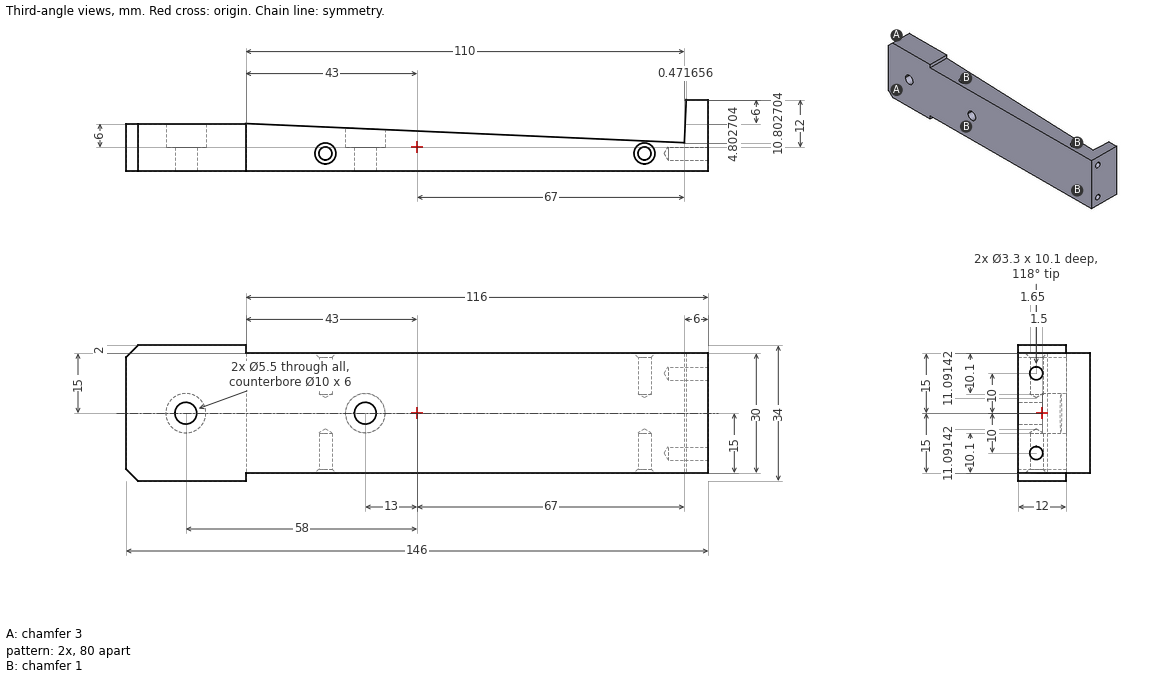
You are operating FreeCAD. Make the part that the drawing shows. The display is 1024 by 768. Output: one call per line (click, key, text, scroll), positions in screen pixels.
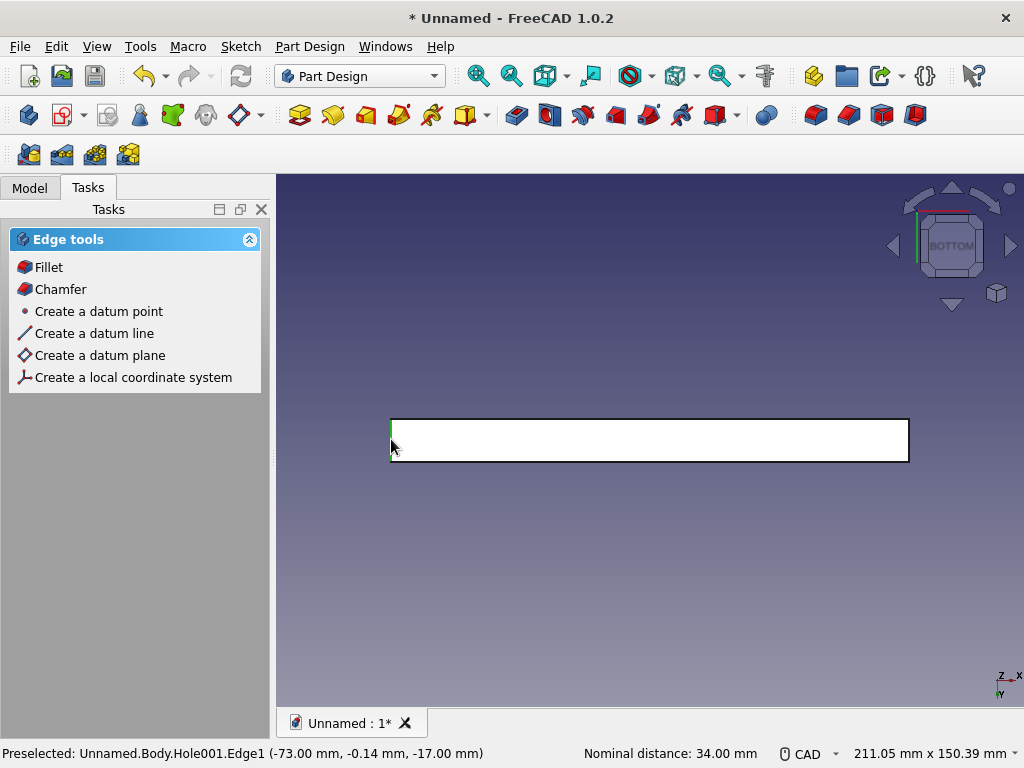
click(849, 116)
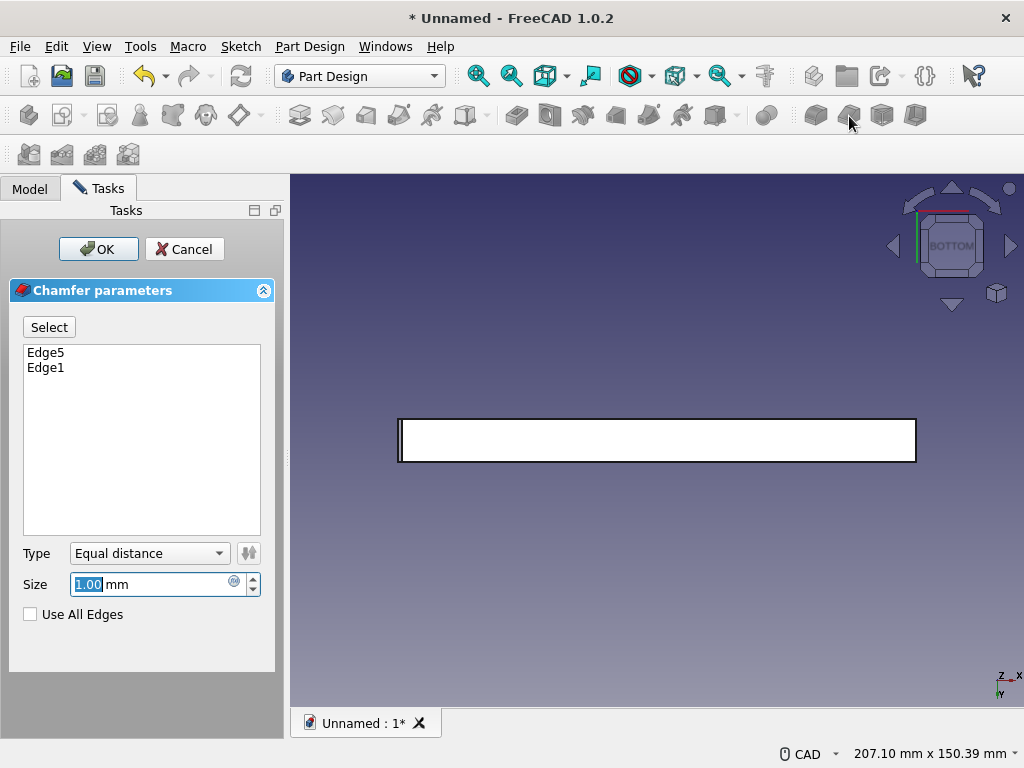
text(3)
key(Tab)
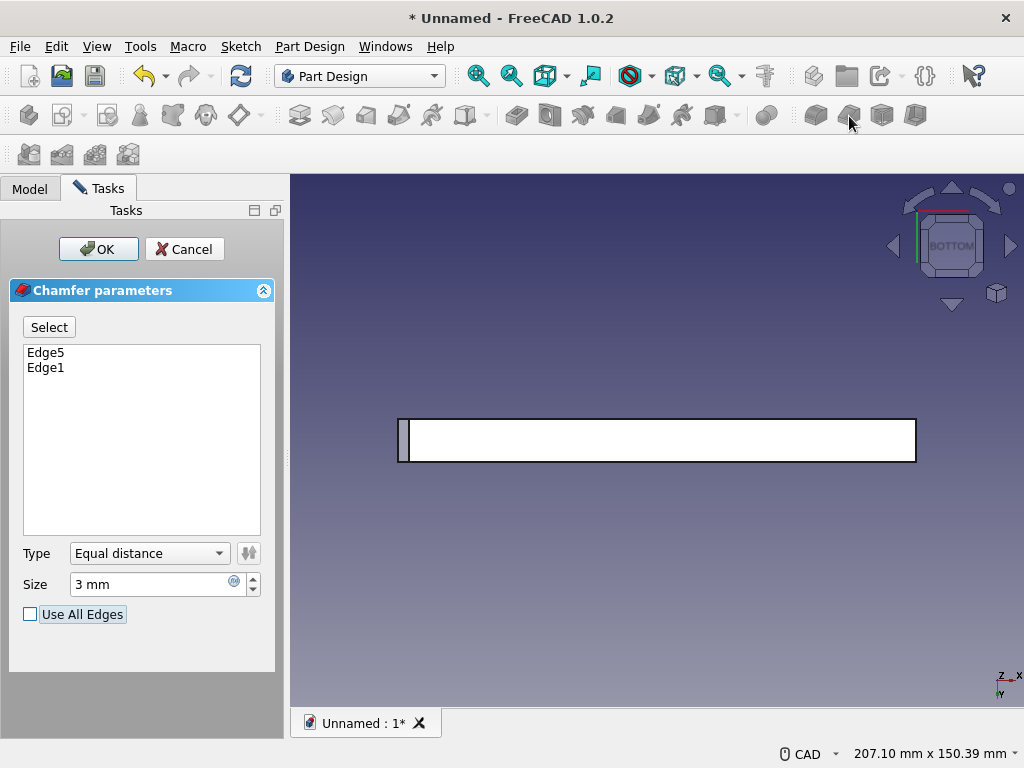
click(99, 249)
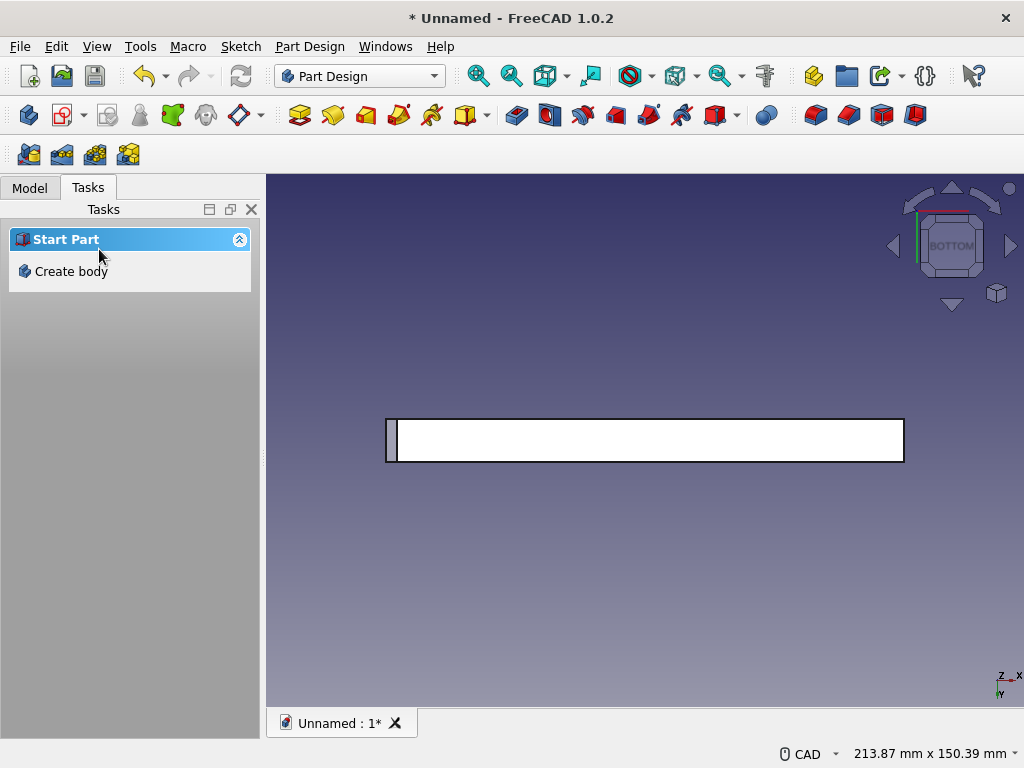
key(4)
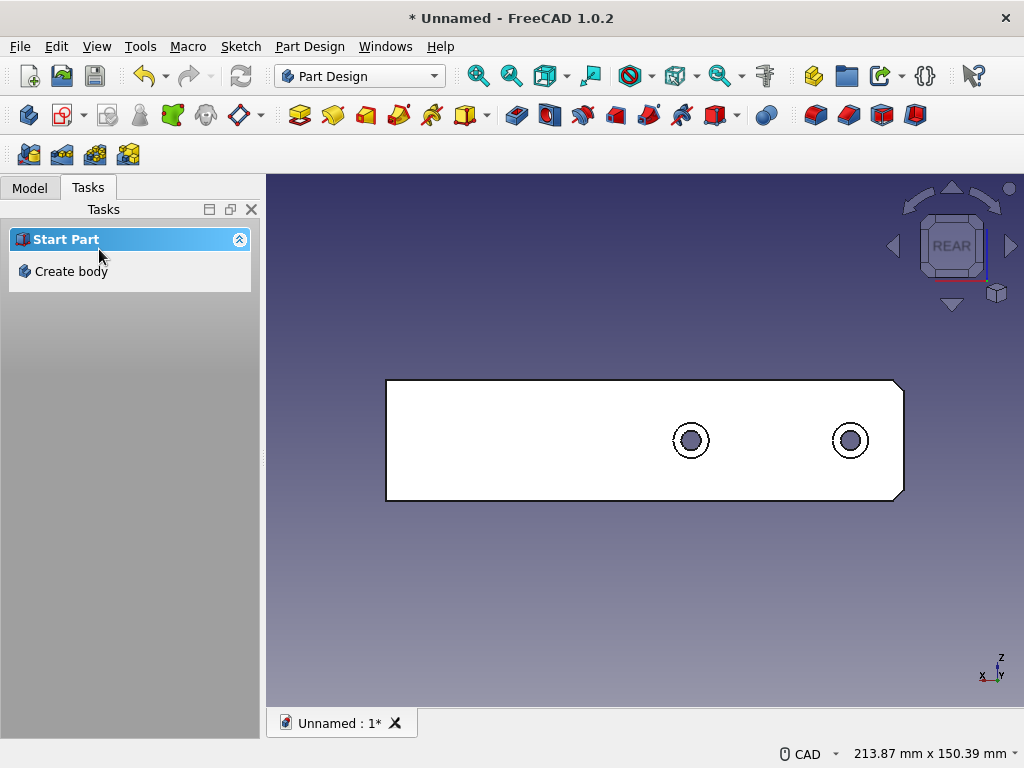
click(497, 439)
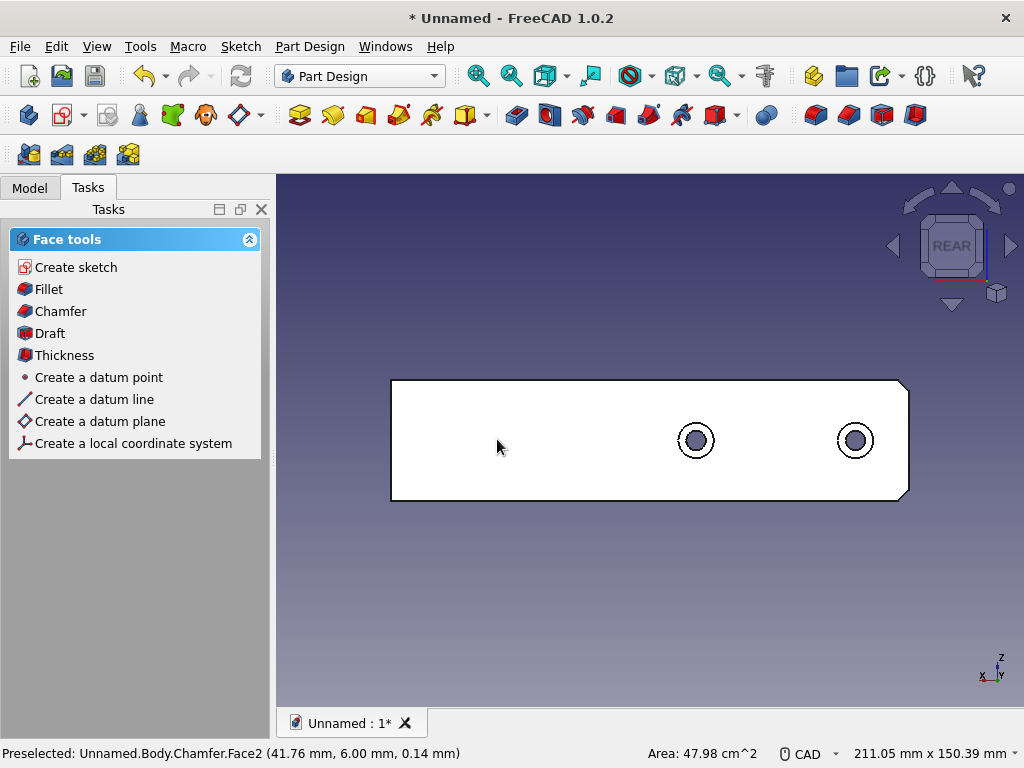
click(62, 116)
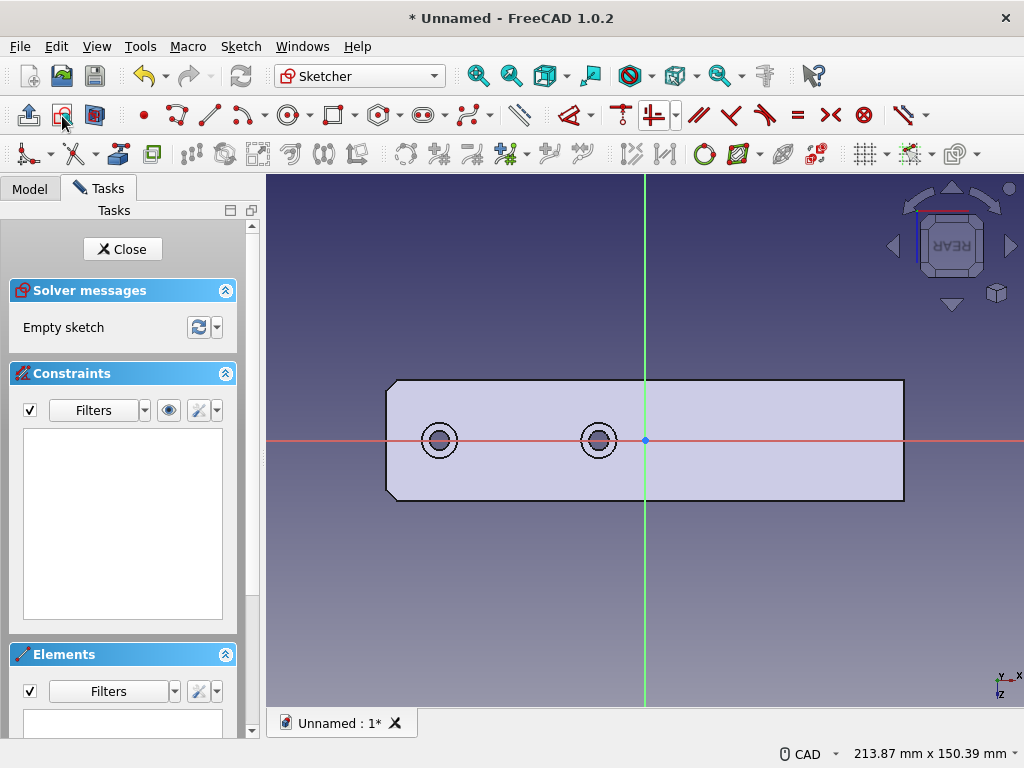
scroll(294, 440, down, 1)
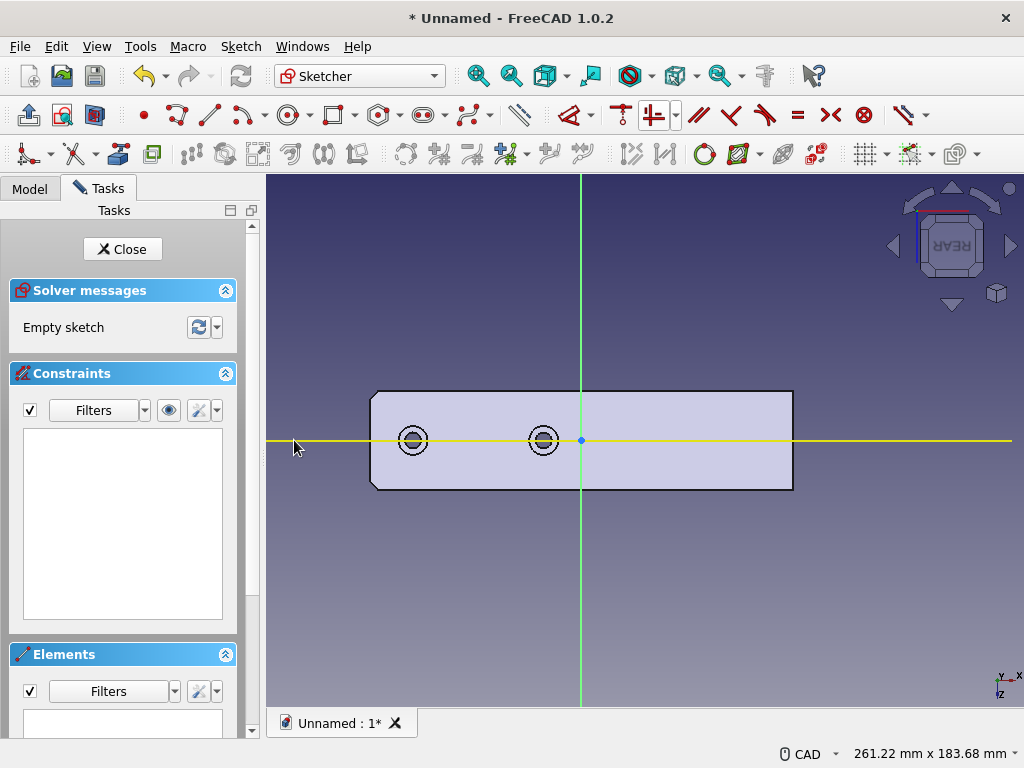
click(332, 116)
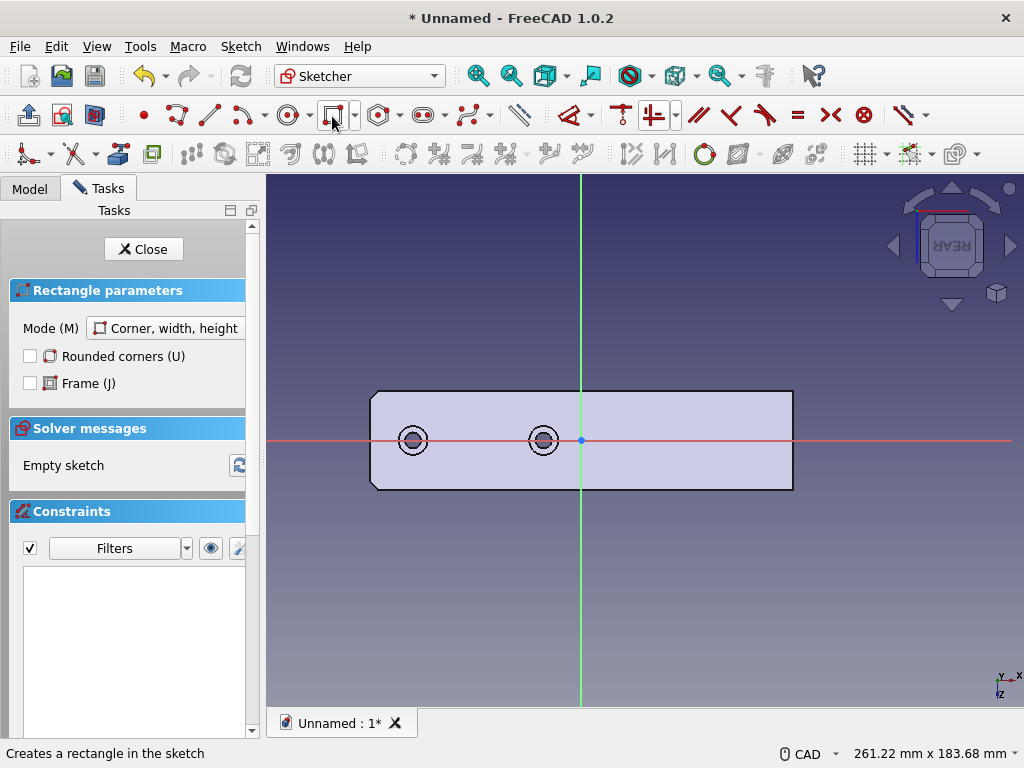
scroll(457, 484, up, 6)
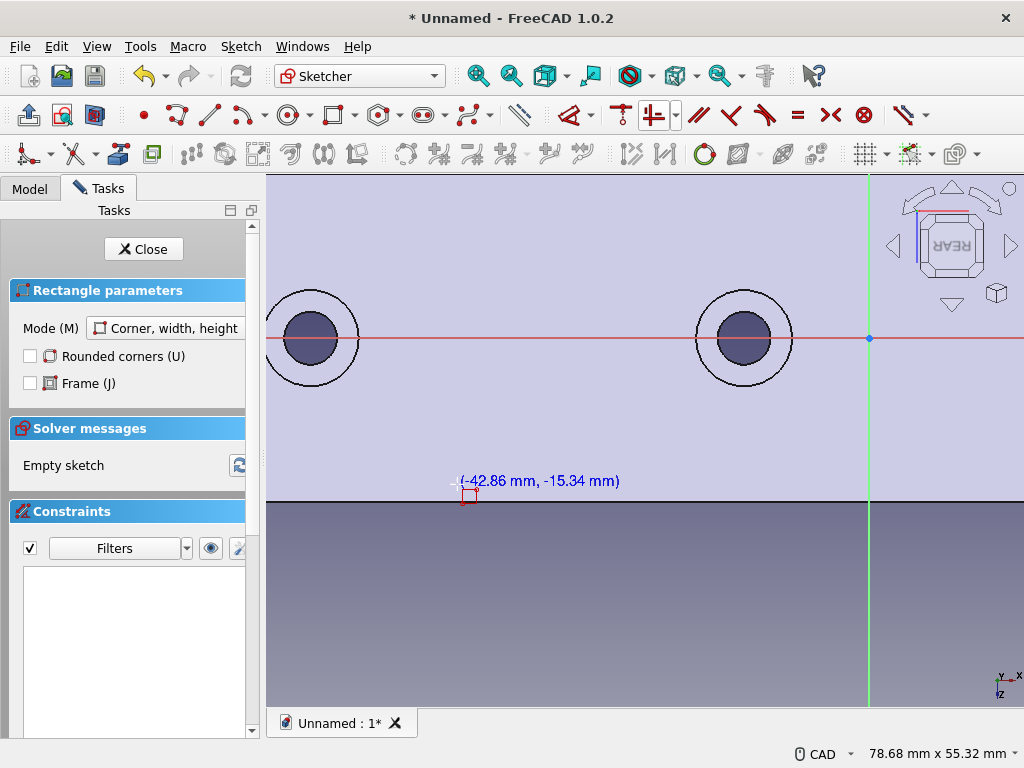
click(455, 483)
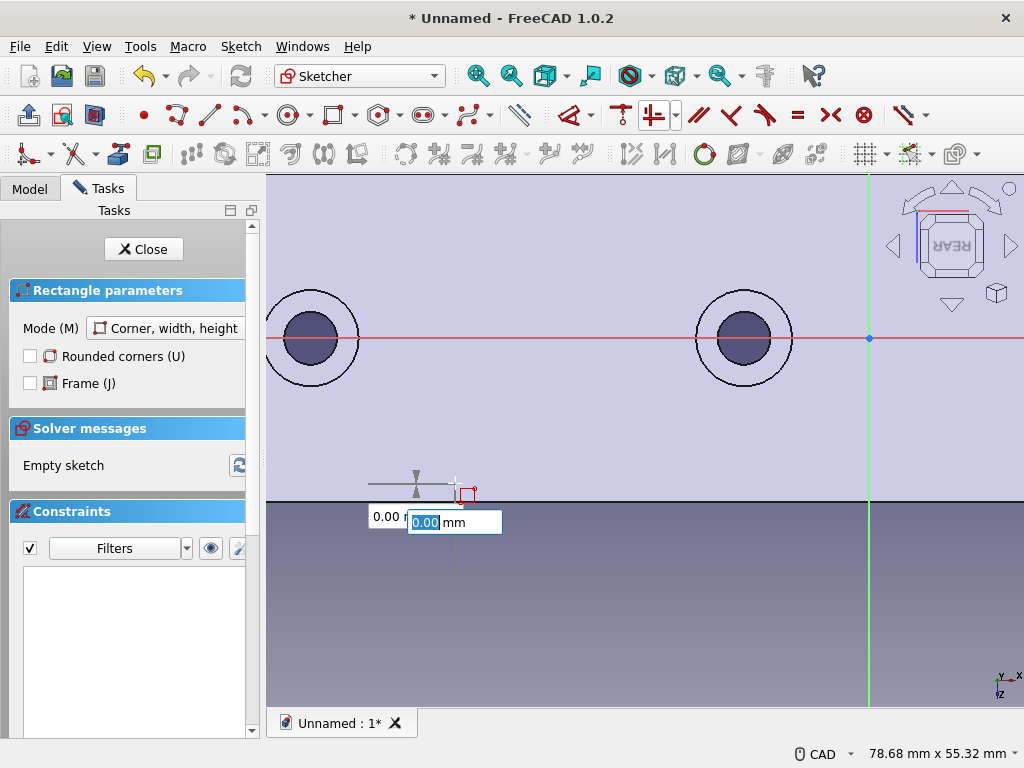
scroll(322, 500, down, 5)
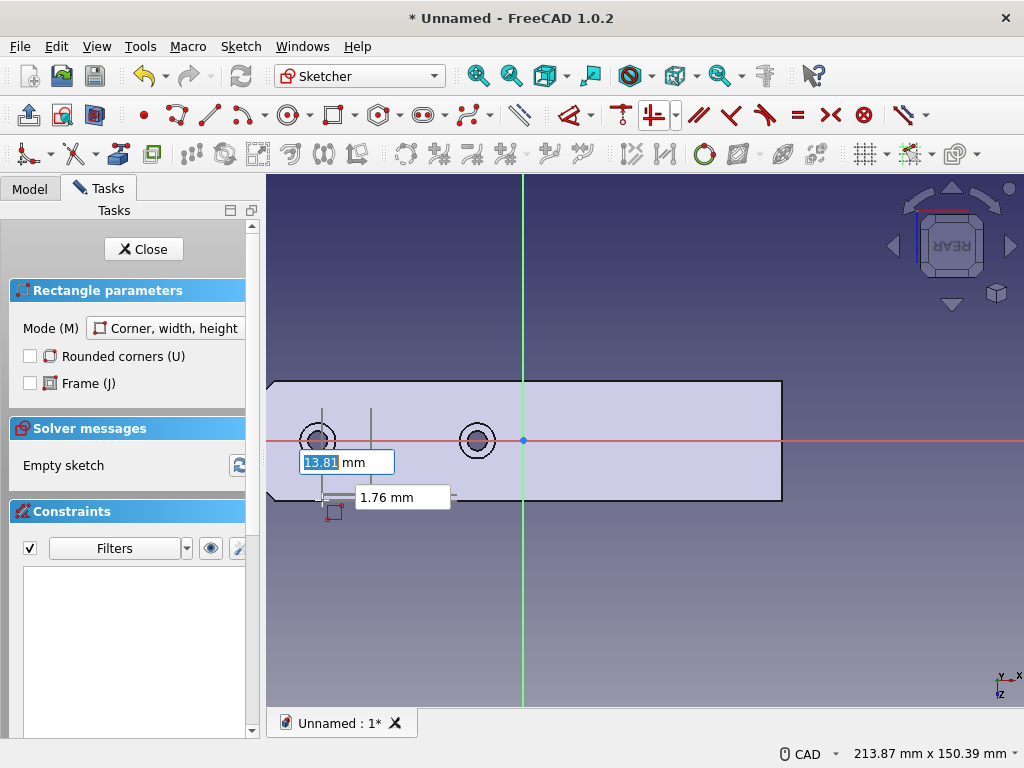
click(782, 501)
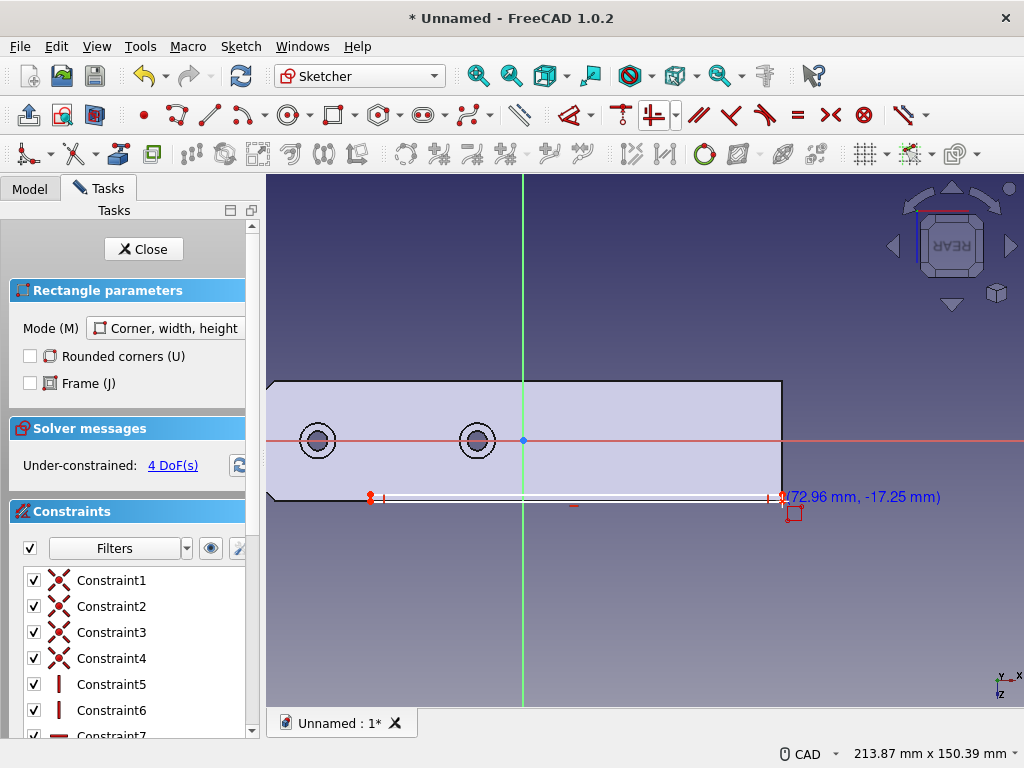
scroll(371, 381, up, 5)